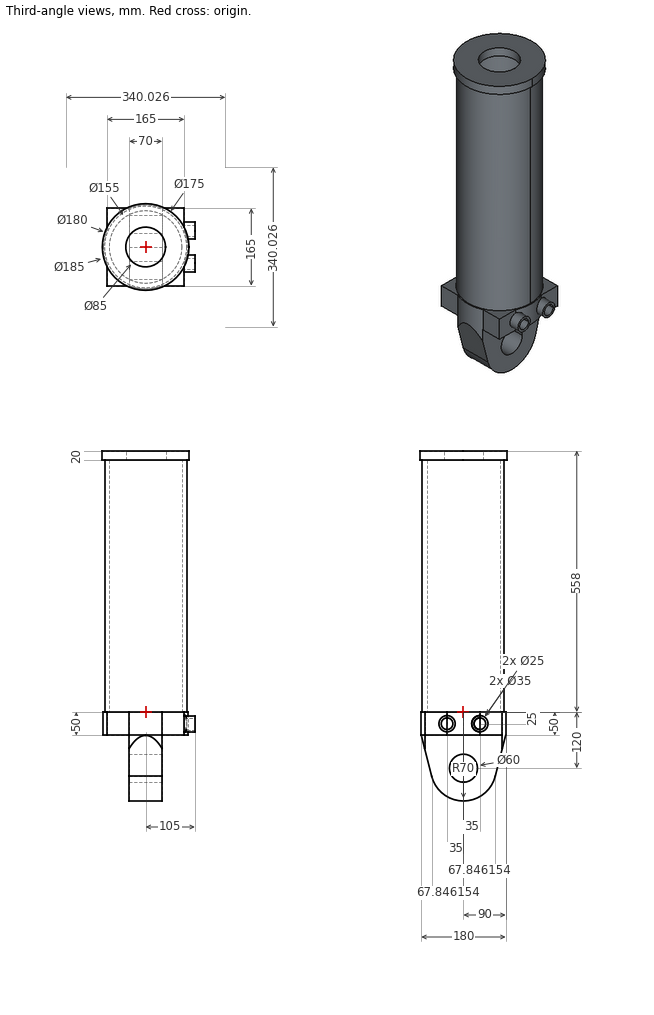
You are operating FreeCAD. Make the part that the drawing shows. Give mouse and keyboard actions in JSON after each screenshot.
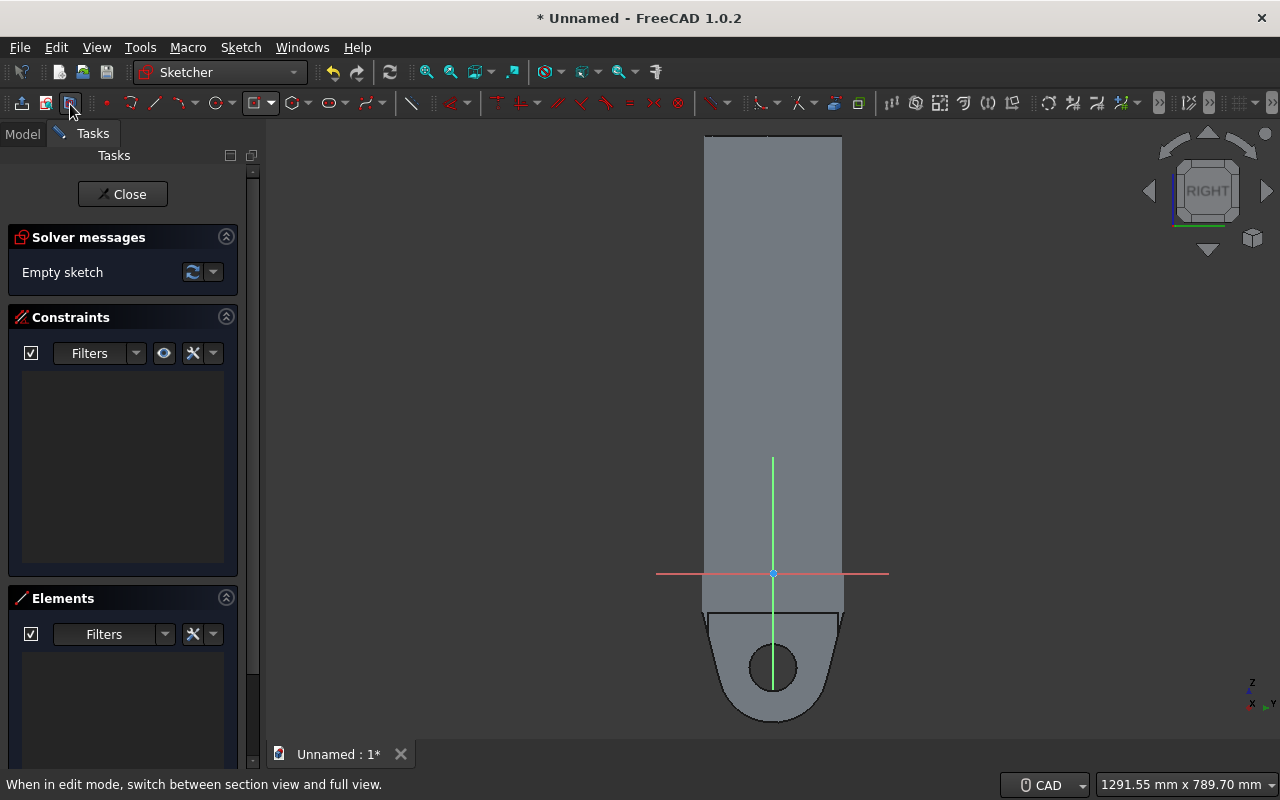
{"action": "scroll", "coordinate": [784, 616], "scroll_direction": "up", "scroll_amount": 10}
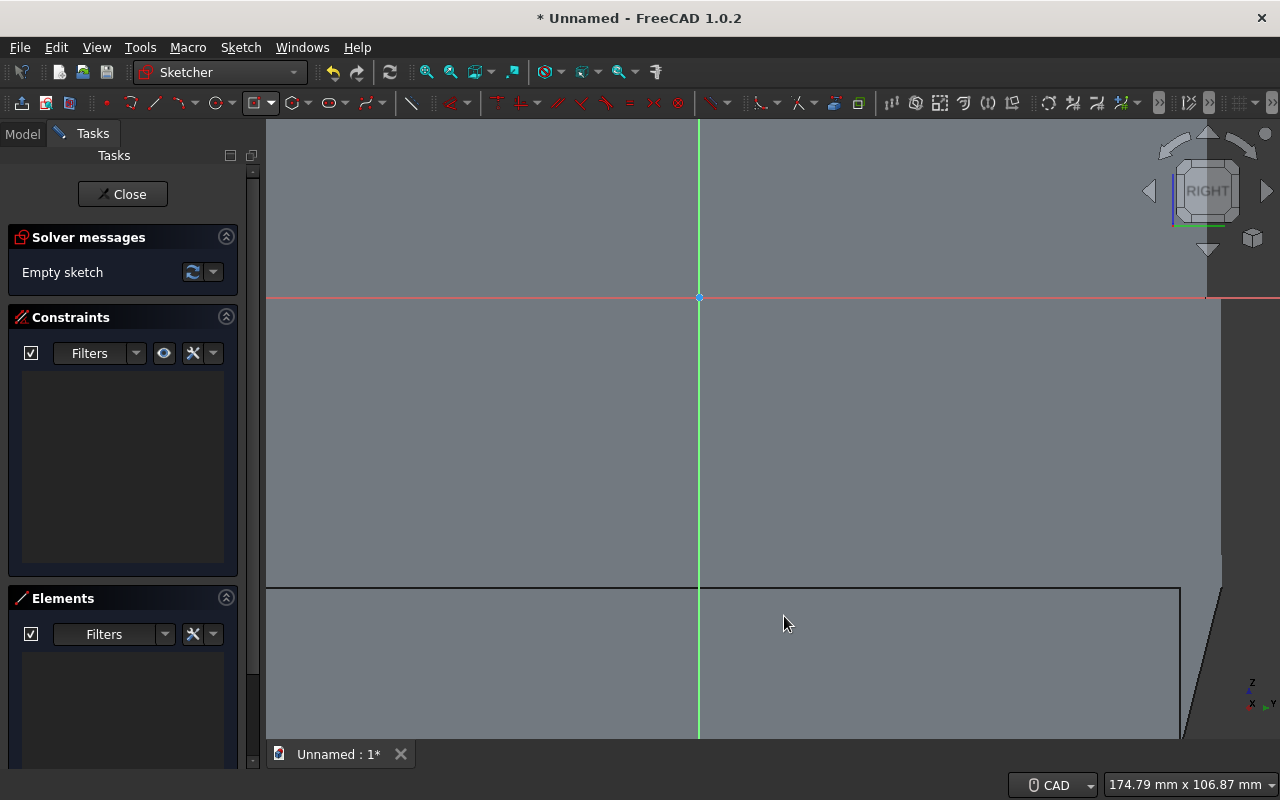
{"action": "left_click", "coordinate": [216, 104]}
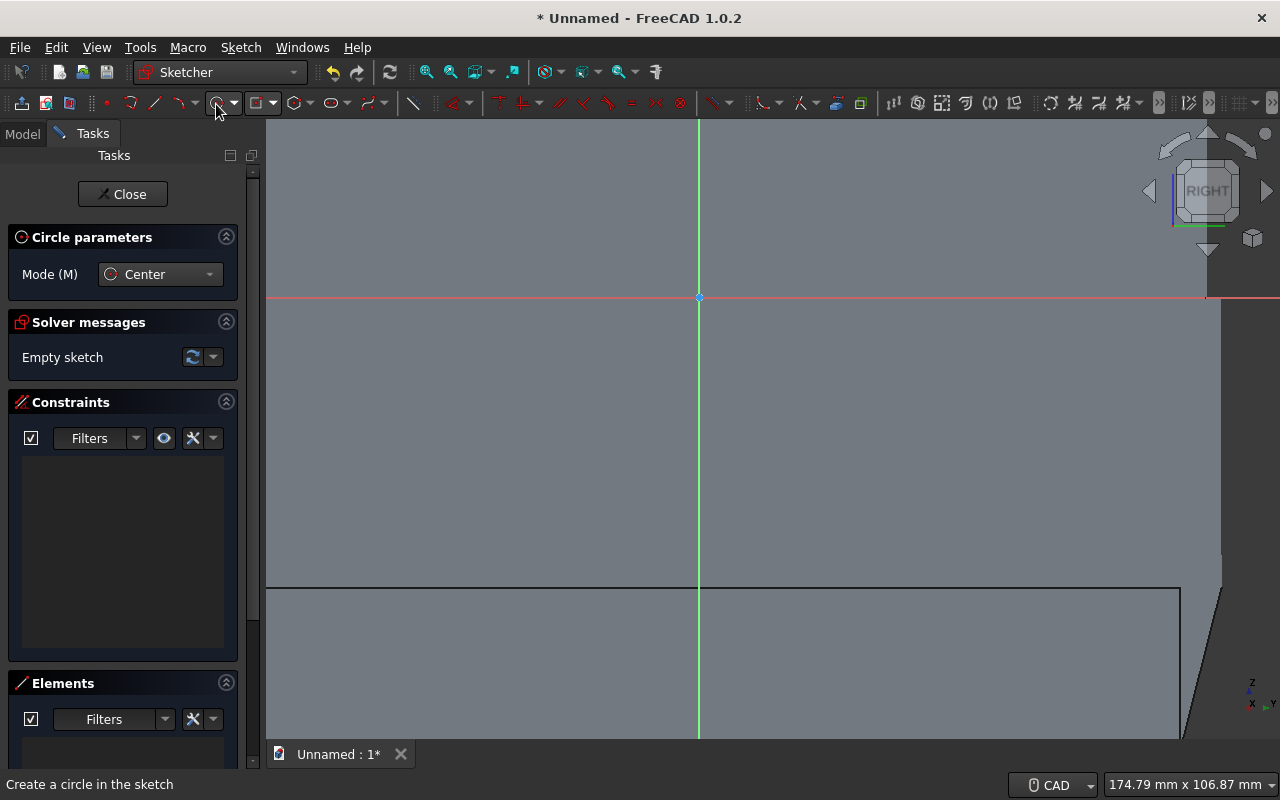
{"action": "left_click", "coordinate": [902, 443]}
{"action": "left_click", "coordinate": [974, 371]}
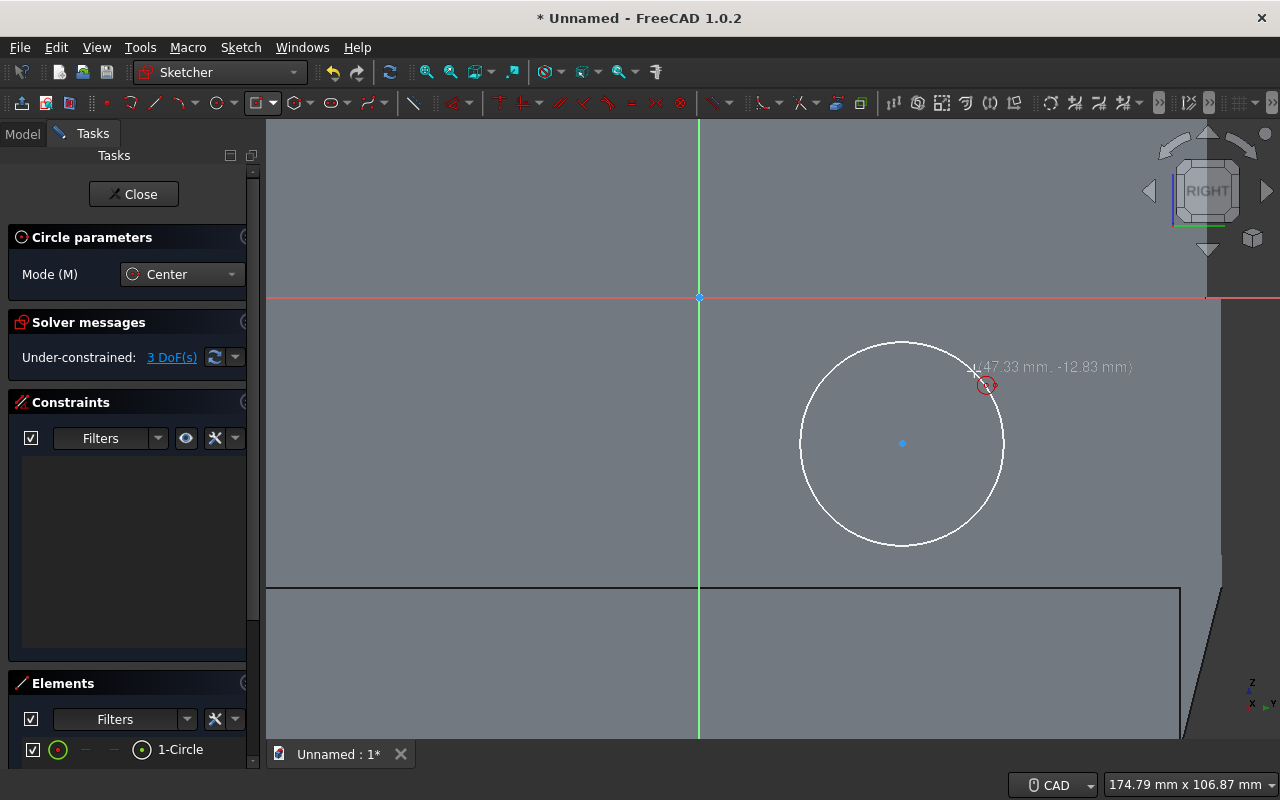
{"action": "left_click", "coordinate": [496, 443]}
{"action": "left_click", "coordinate": [568, 371]}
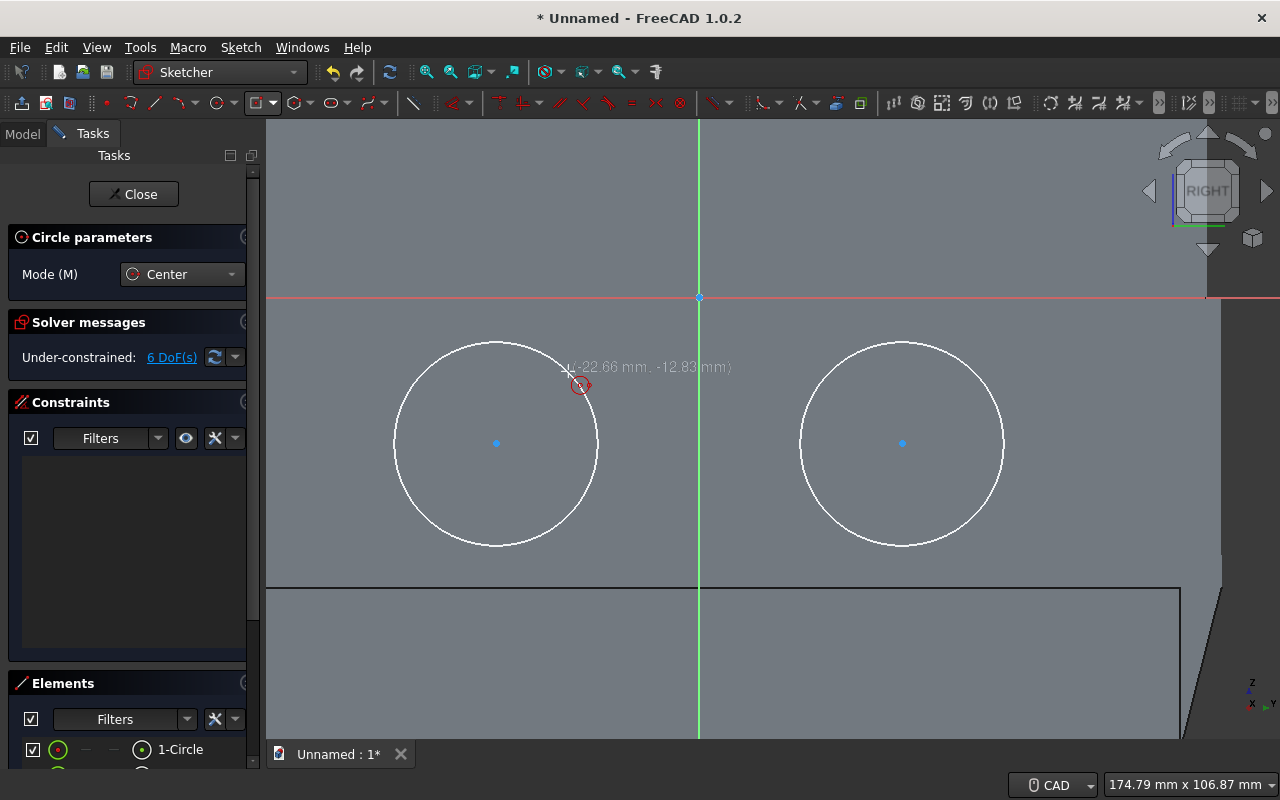
{"action": "left_click", "coordinate": [902, 444]}
{"action": "left_click", "coordinate": [954, 391]}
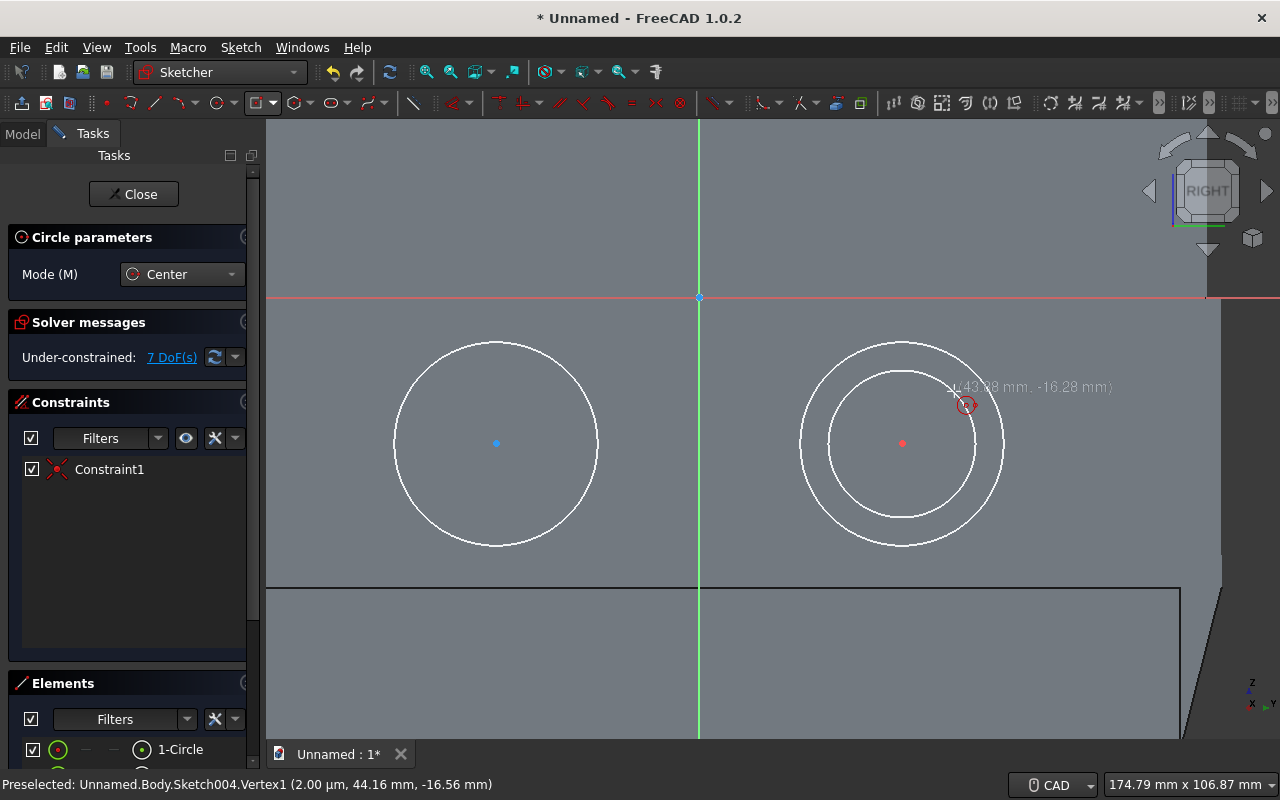
{"action": "left_click", "coordinate": [496, 444]}
{"action": "left_click", "coordinate": [548, 391]}
{"action": "key", "text": "Escape"}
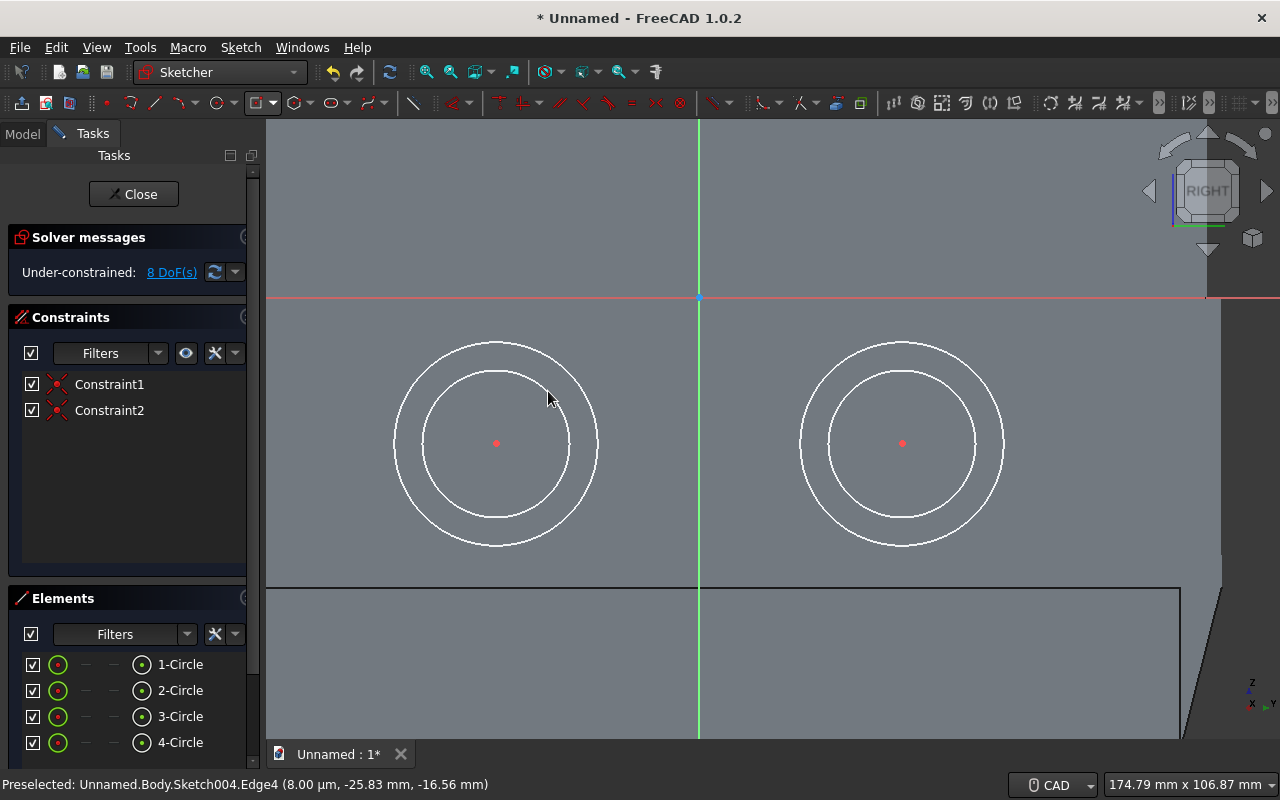
{"action": "left_click", "coordinate": [974, 372]}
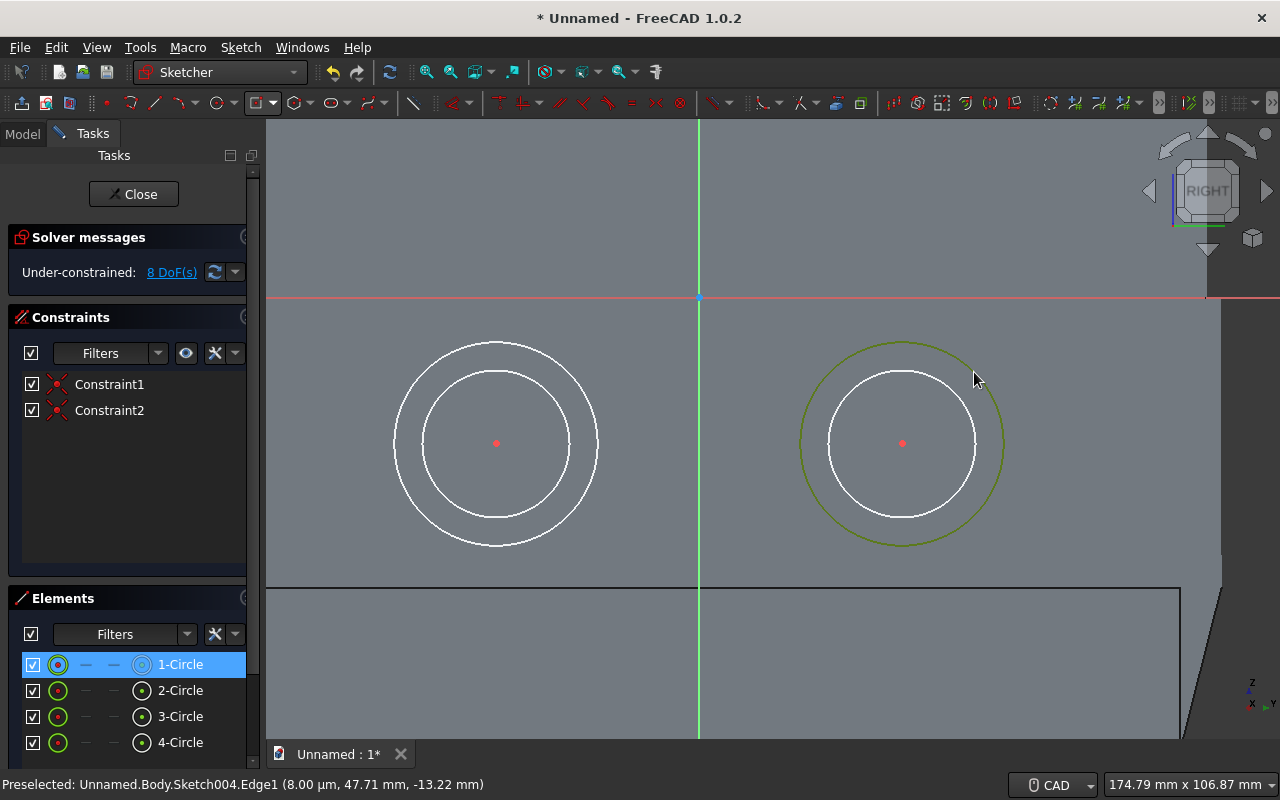
{"action": "left_click", "coordinate": [568, 372]}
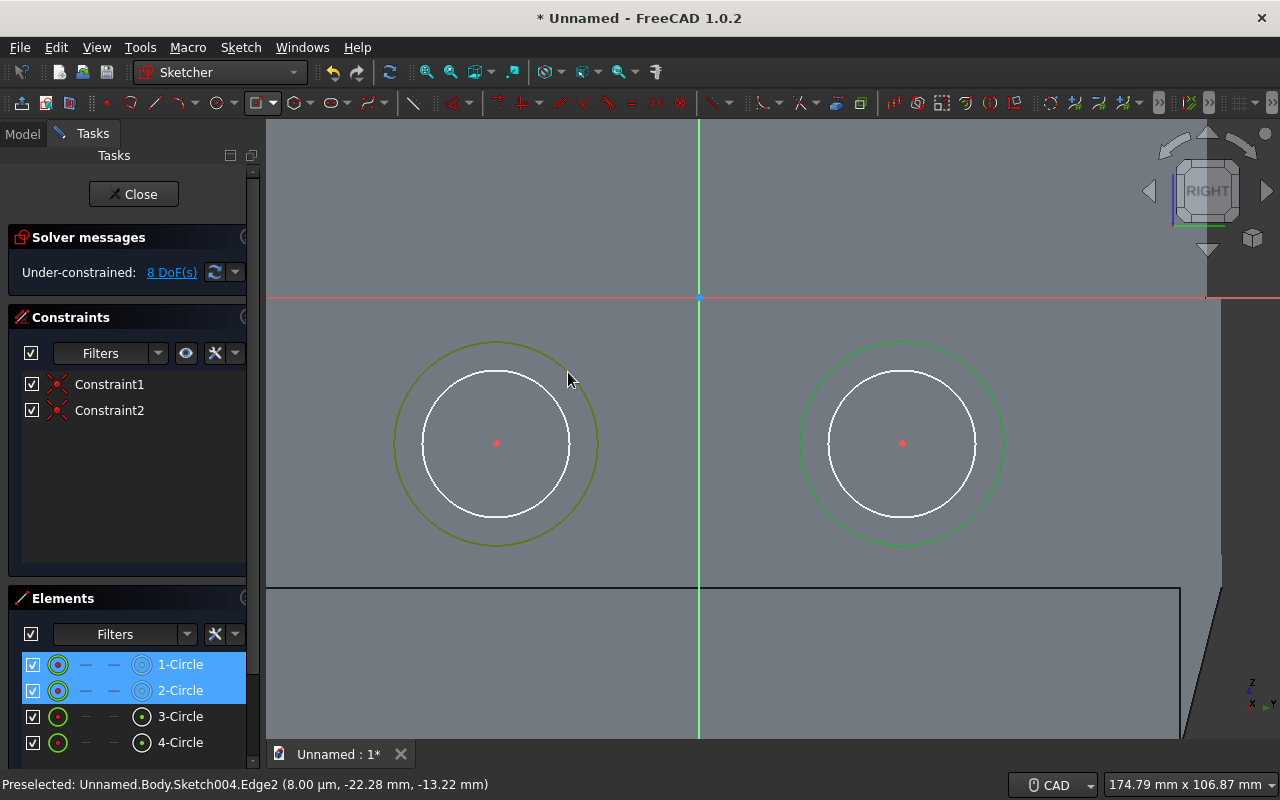
{"action": "left_click", "coordinate": [632, 104]}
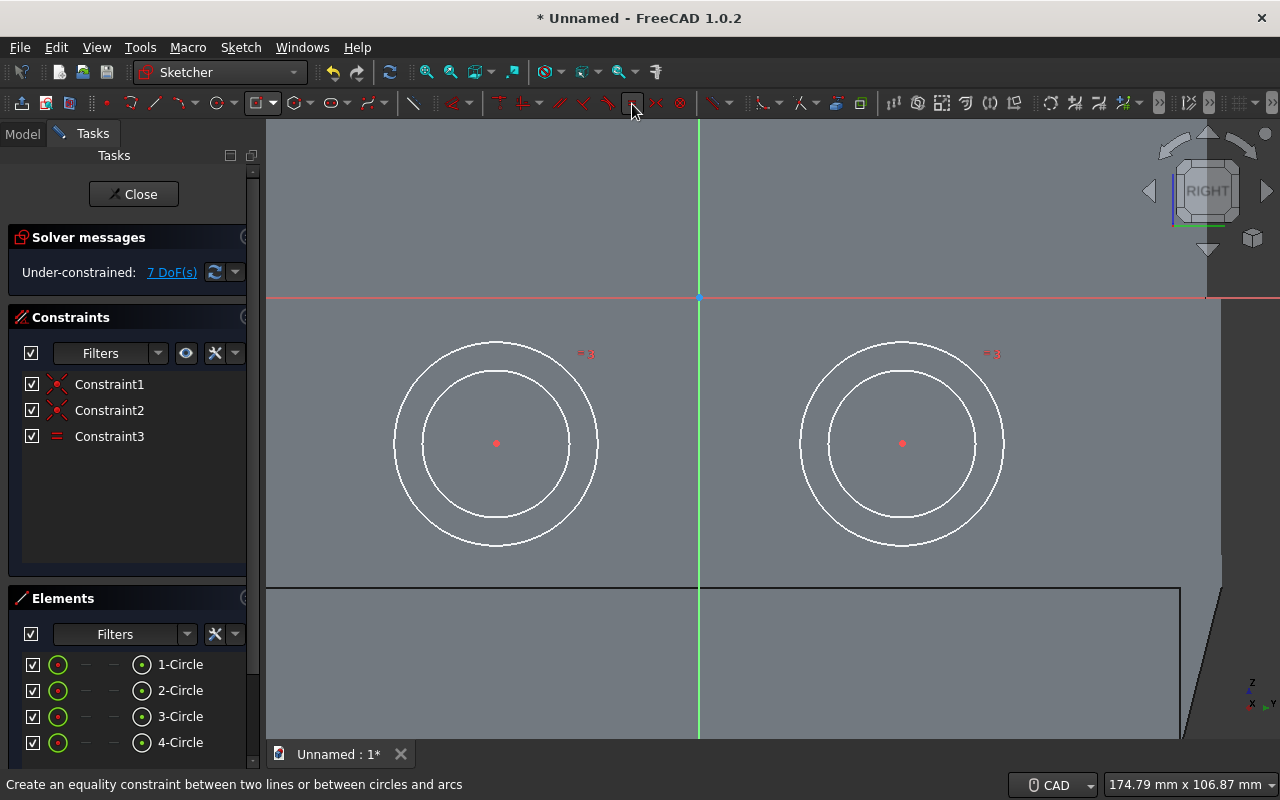
{"action": "left_click", "coordinate": [954, 392]}